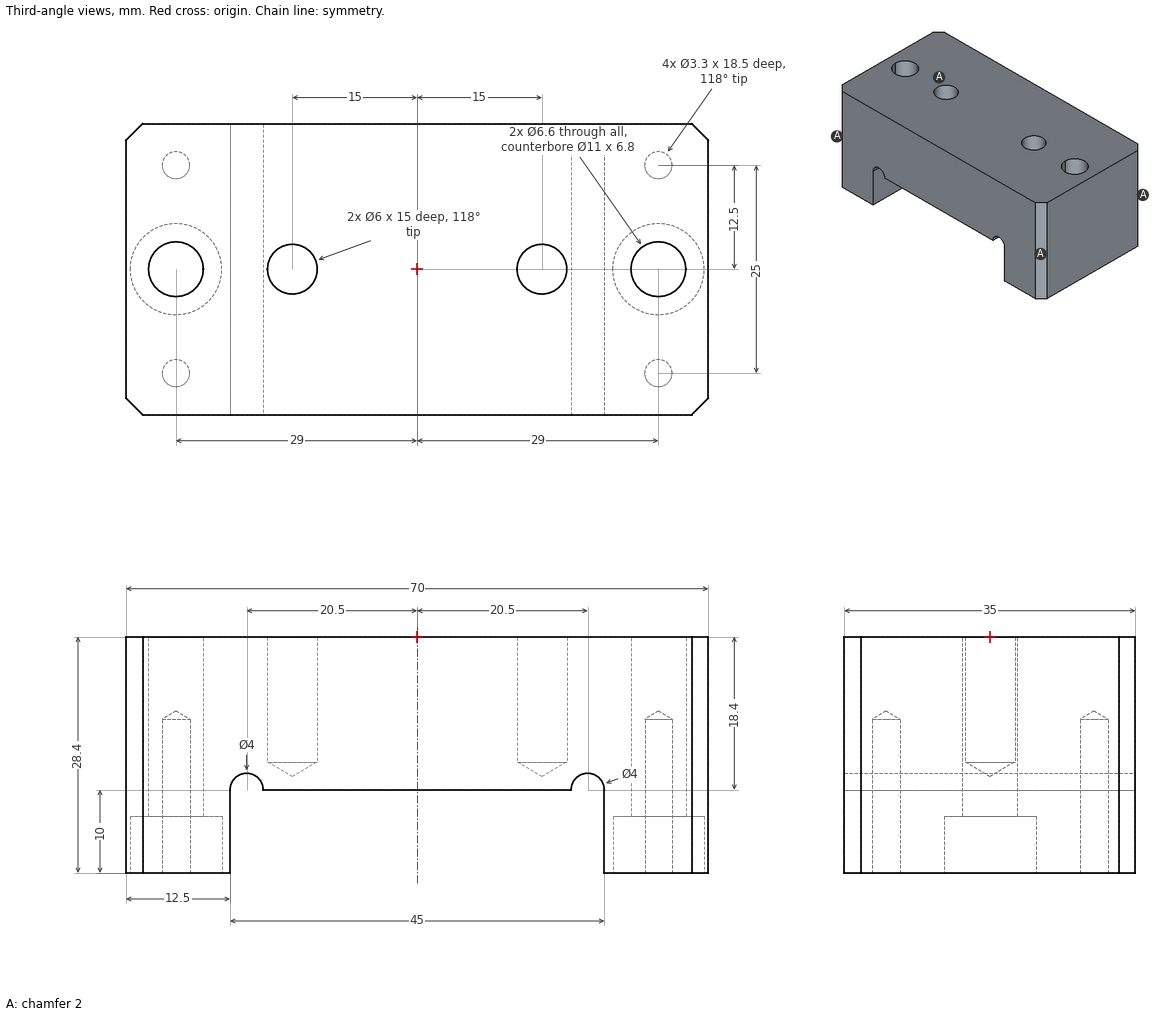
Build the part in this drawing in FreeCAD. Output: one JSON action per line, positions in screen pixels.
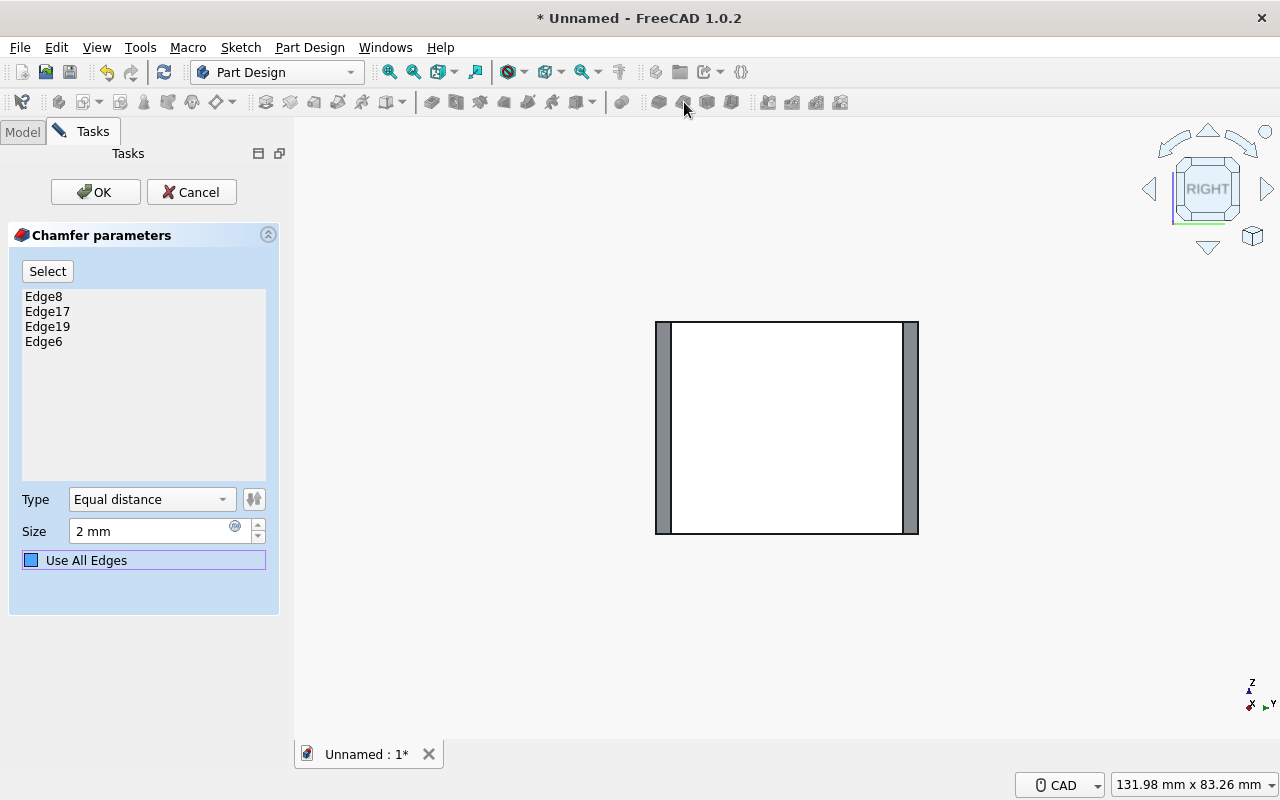
{"action": "left_click", "coordinate": [96, 192]}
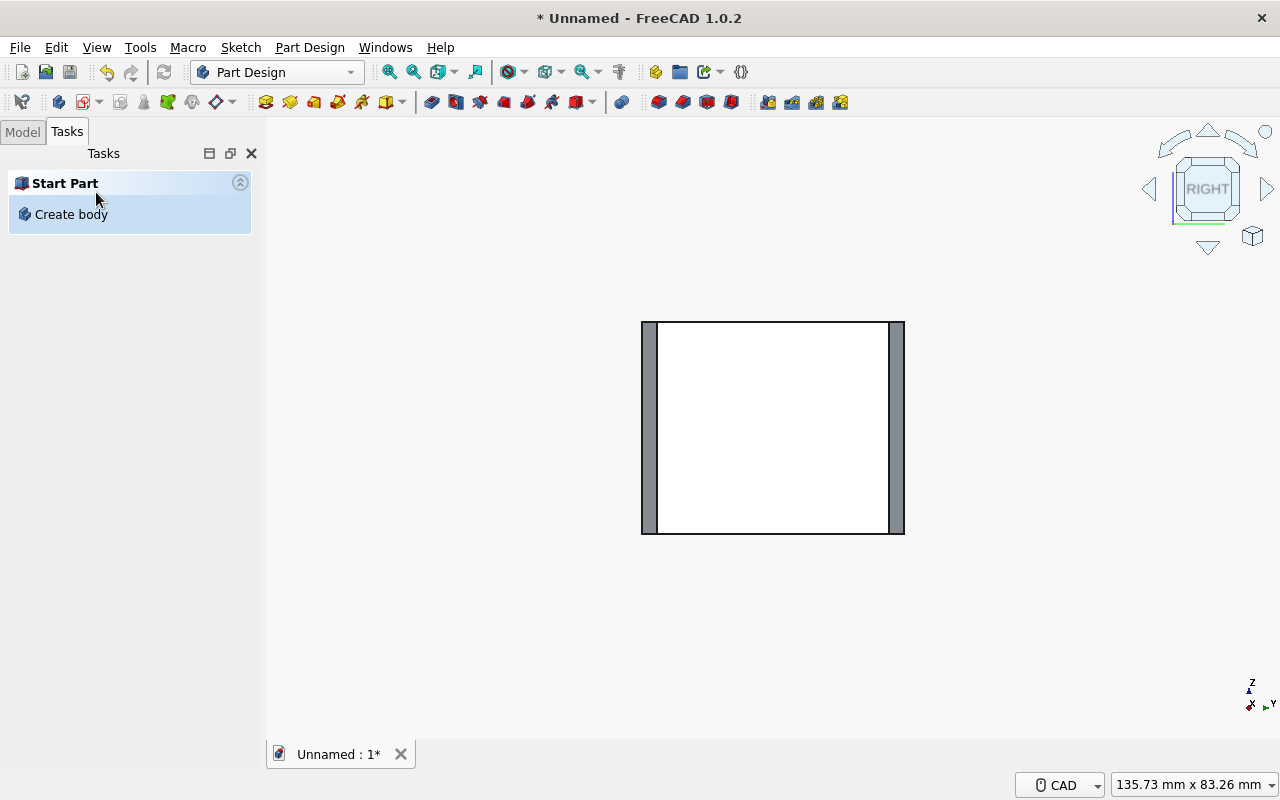
{"action": "key", "text": "v f"}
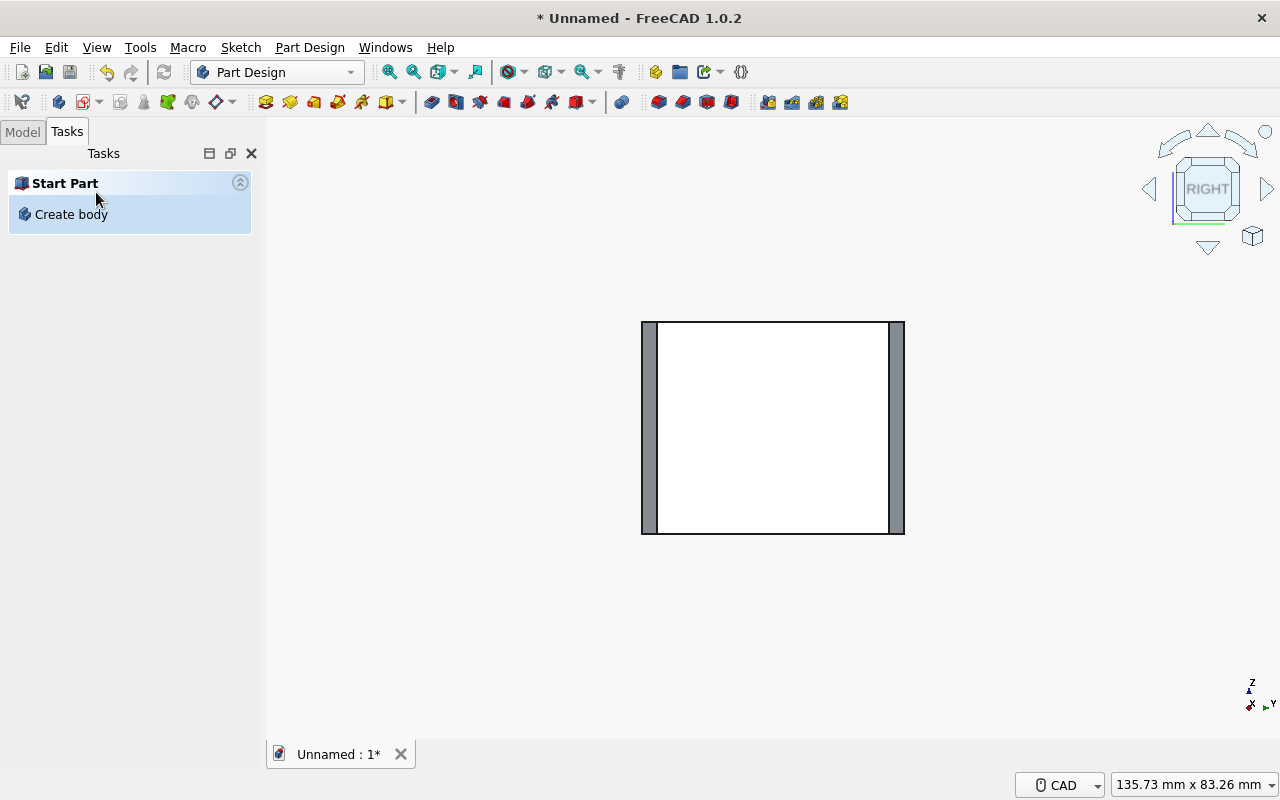
{"action": "key", "text": "0"}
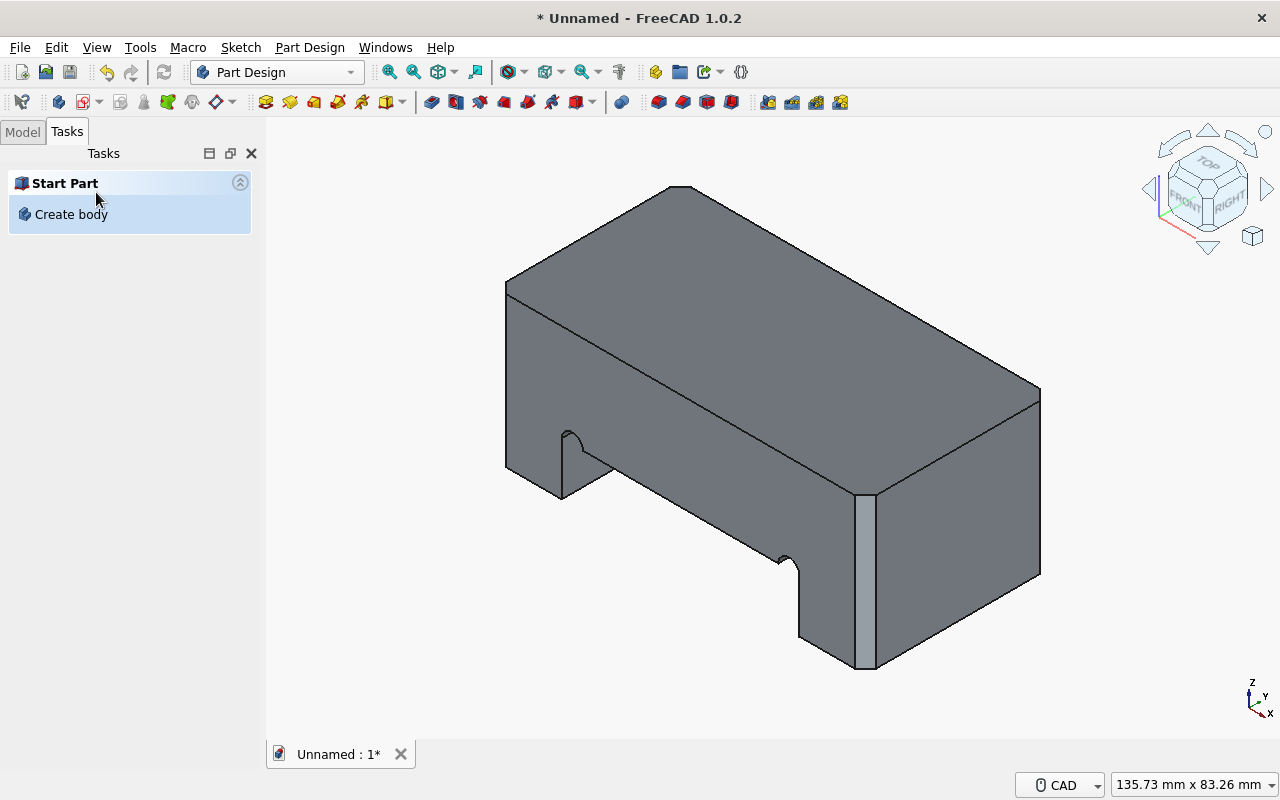
{"action": "left_click", "coordinate": [826, 371]}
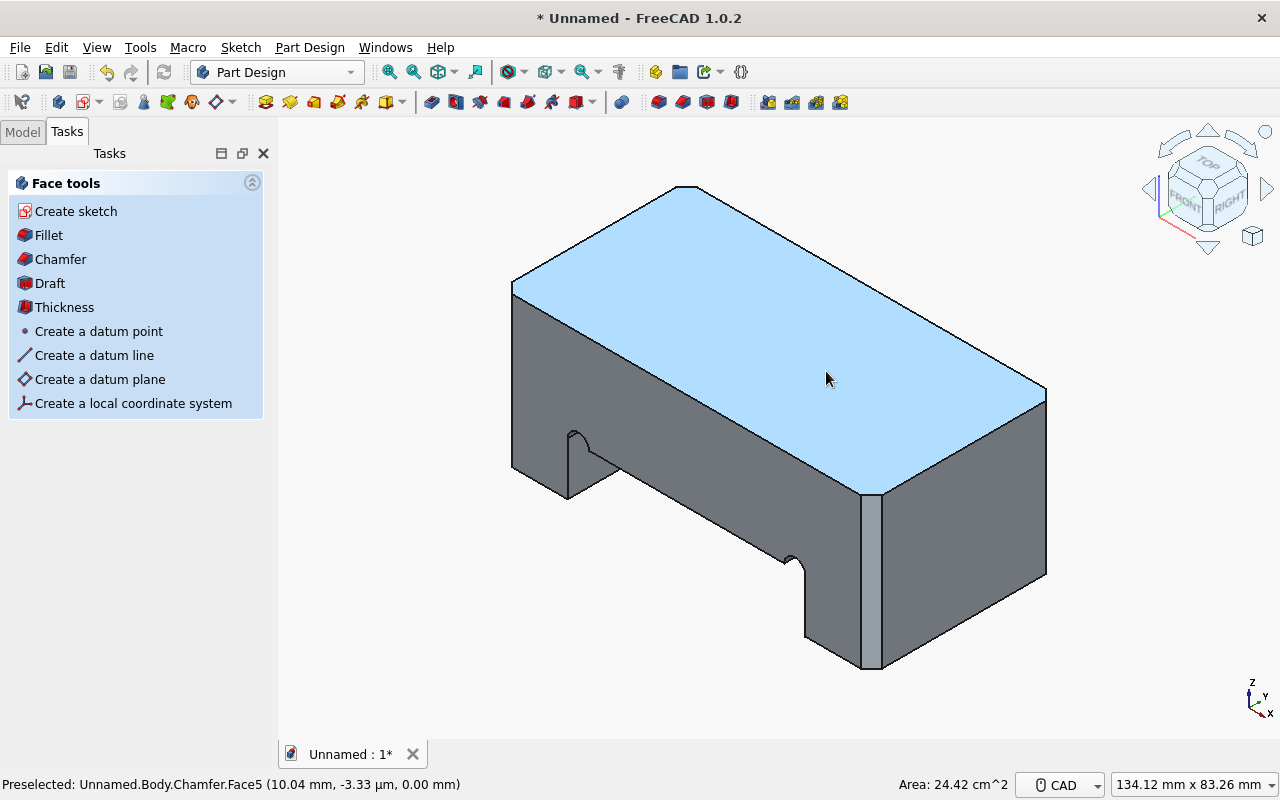
{"action": "left_click", "coordinate": [84, 102]}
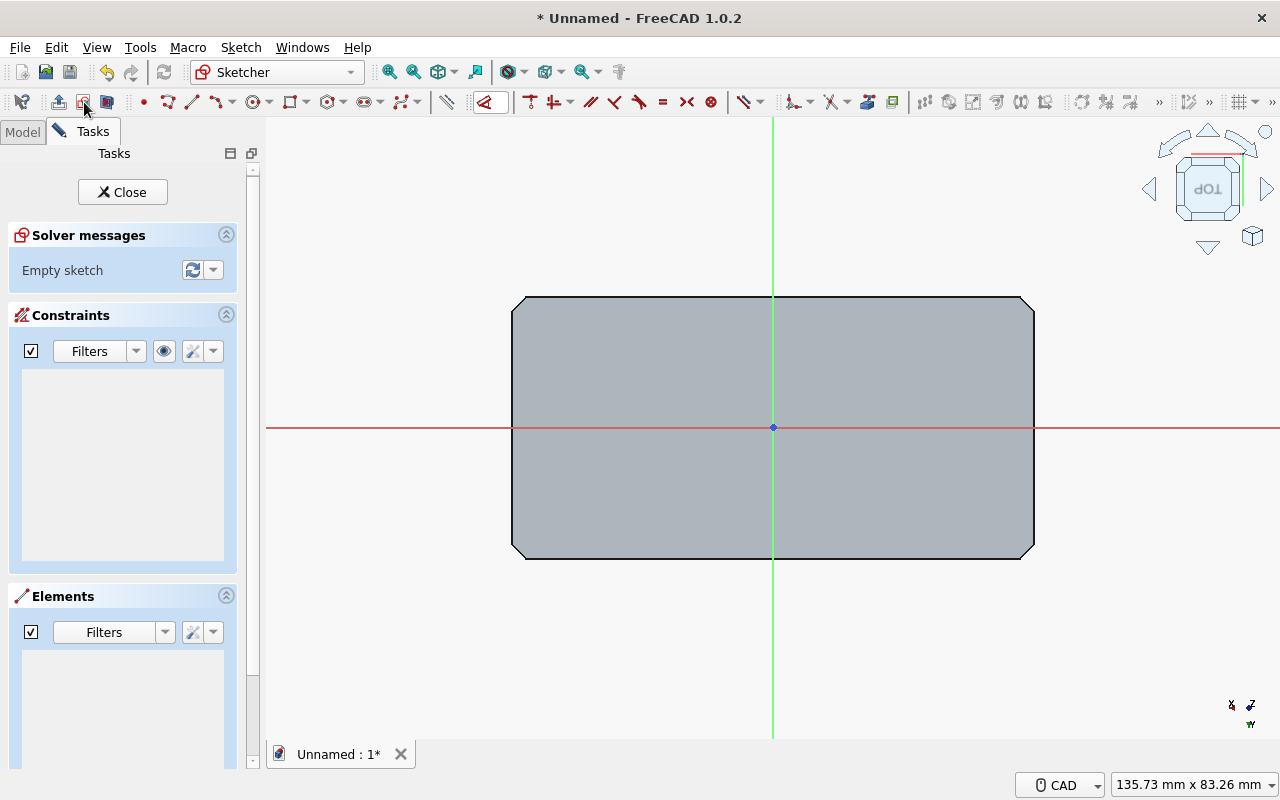
{"action": "scroll", "coordinate": [829, 428], "scroll_direction": "up", "scroll_amount": 4}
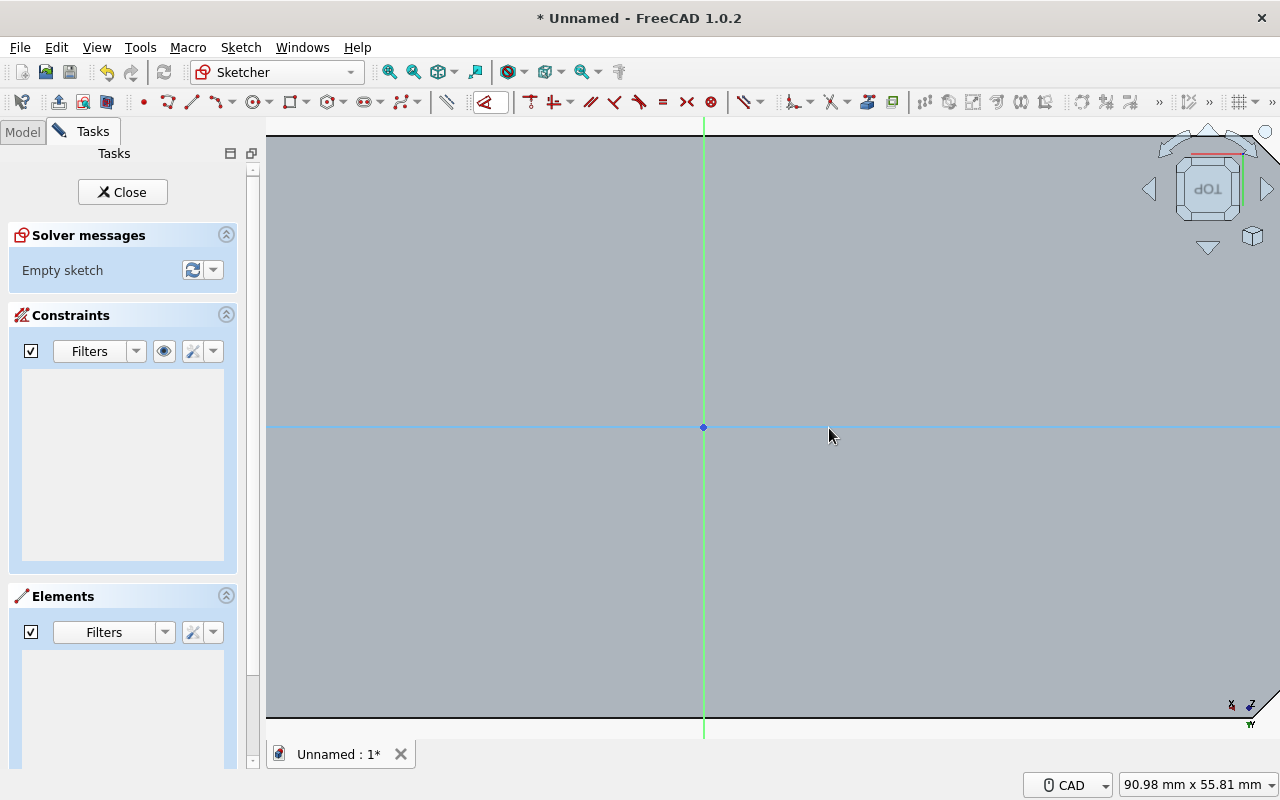
{"action": "key", "text": "g c"}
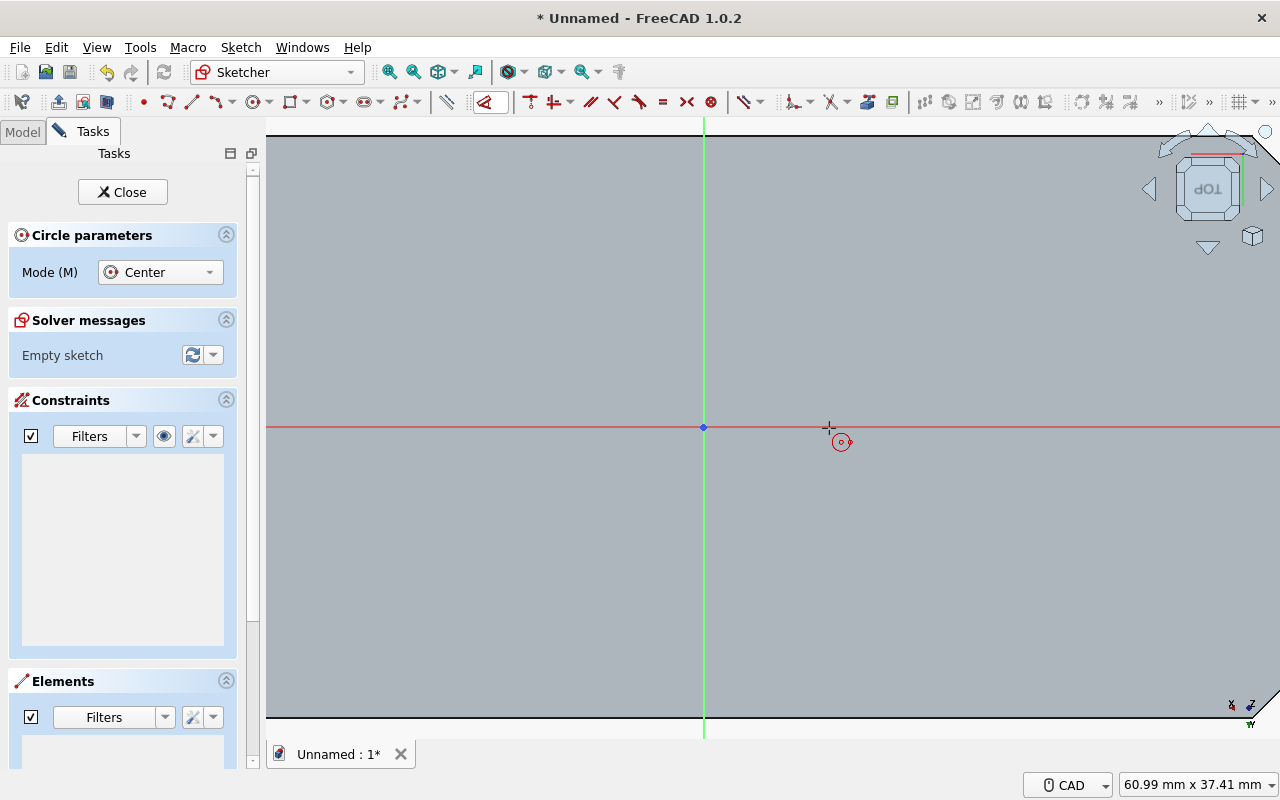
{"action": "left_click", "coordinate": [953, 427]}
{"action": "left_click", "coordinate": [988, 392]}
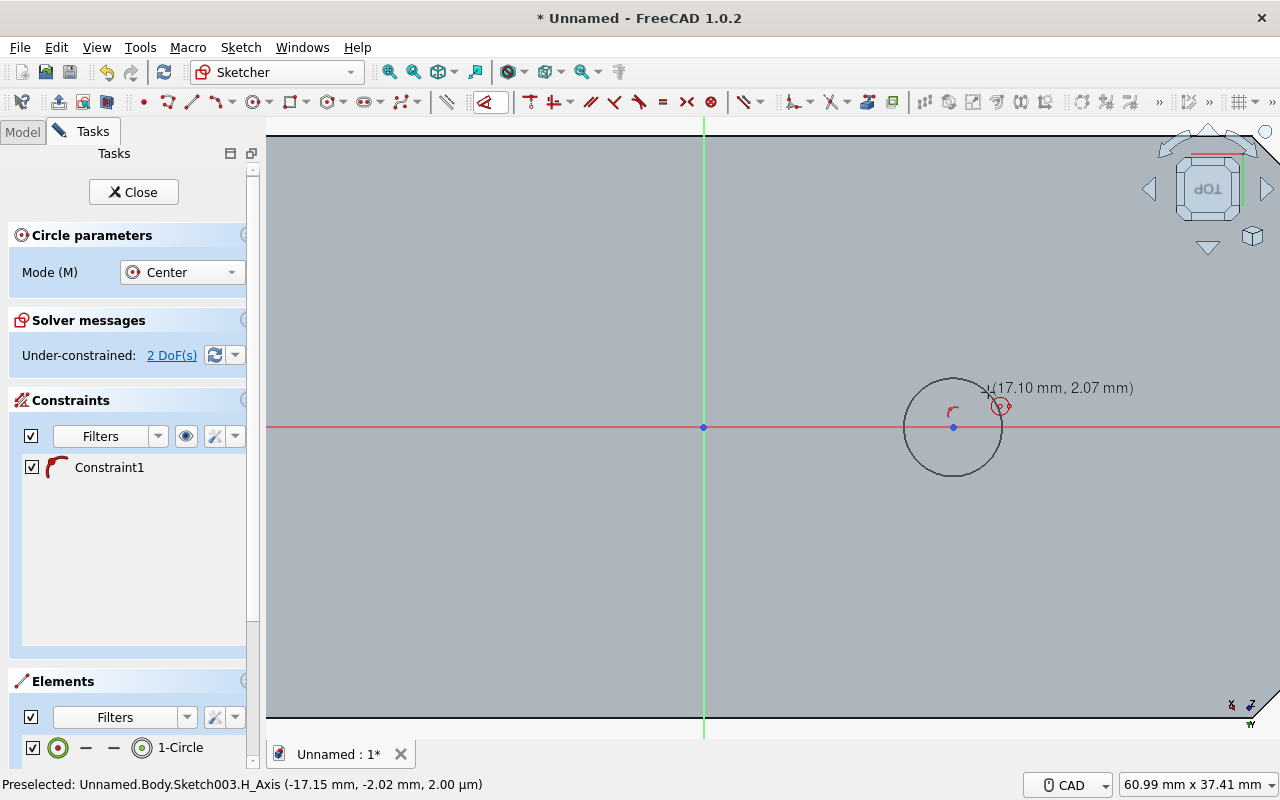
{"action": "left_click", "coordinate": [454, 427]}
{"action": "left_click", "coordinate": [490, 392]}
{"action": "key", "text": "Escape"}